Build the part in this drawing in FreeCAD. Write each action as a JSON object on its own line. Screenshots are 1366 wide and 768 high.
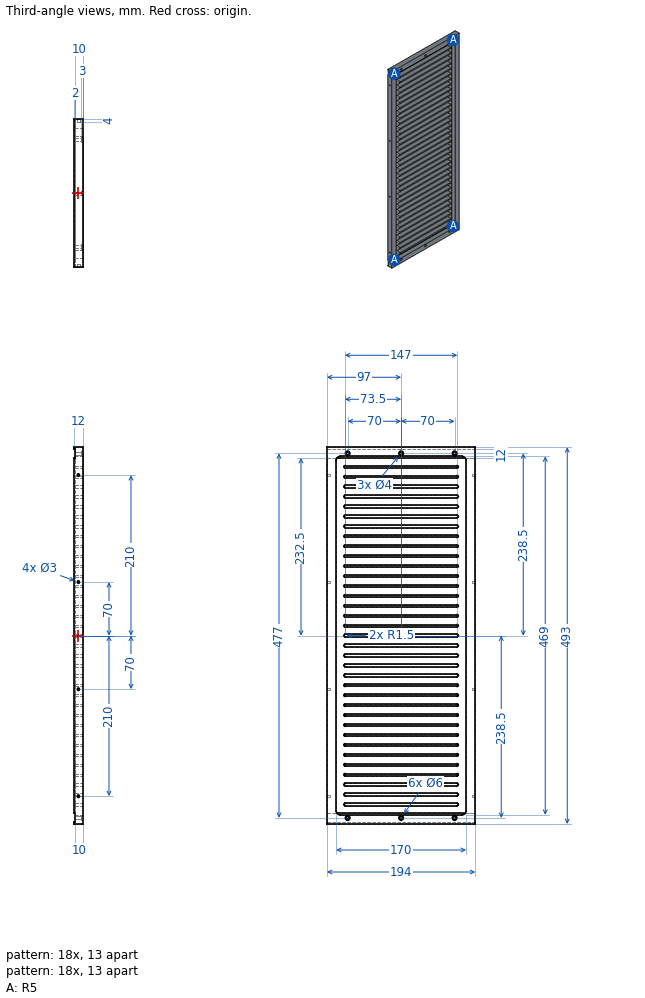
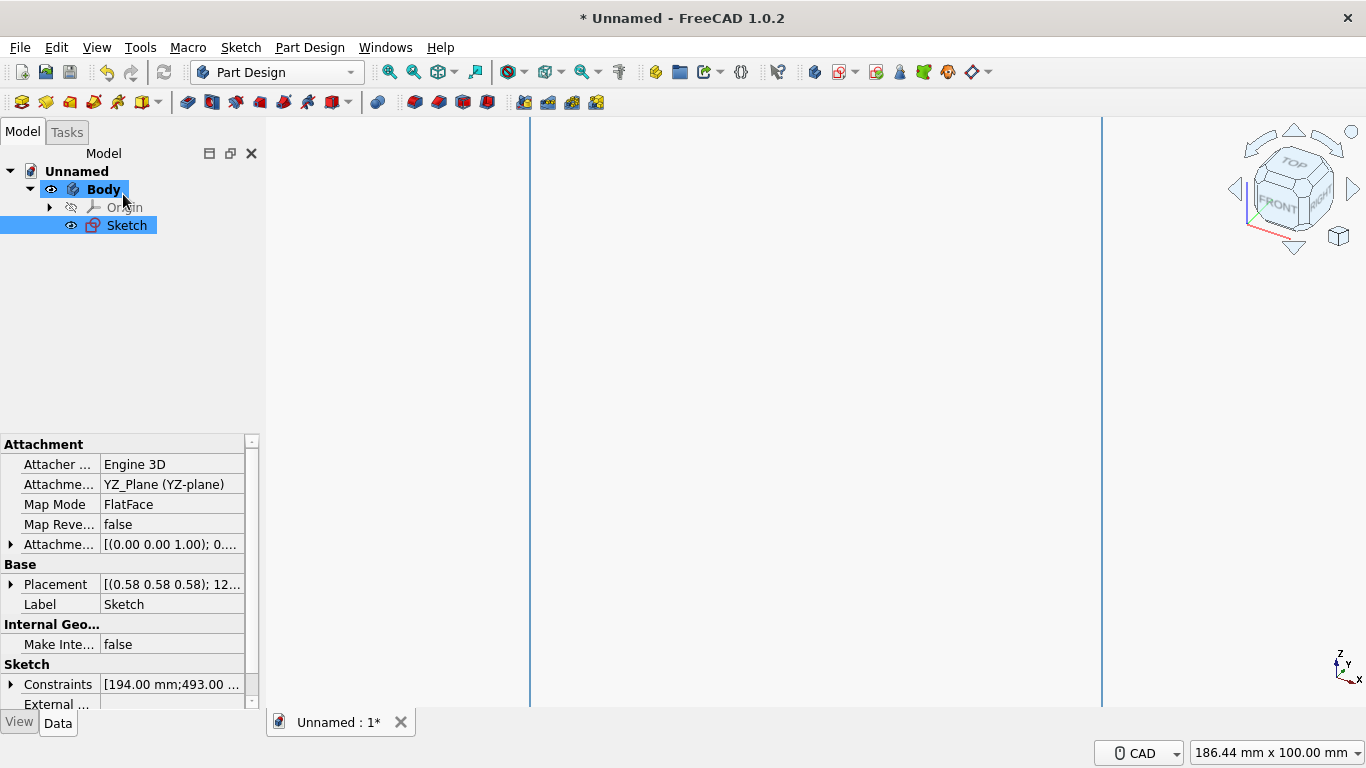
{"action": "left_click", "coordinate": [22, 102]}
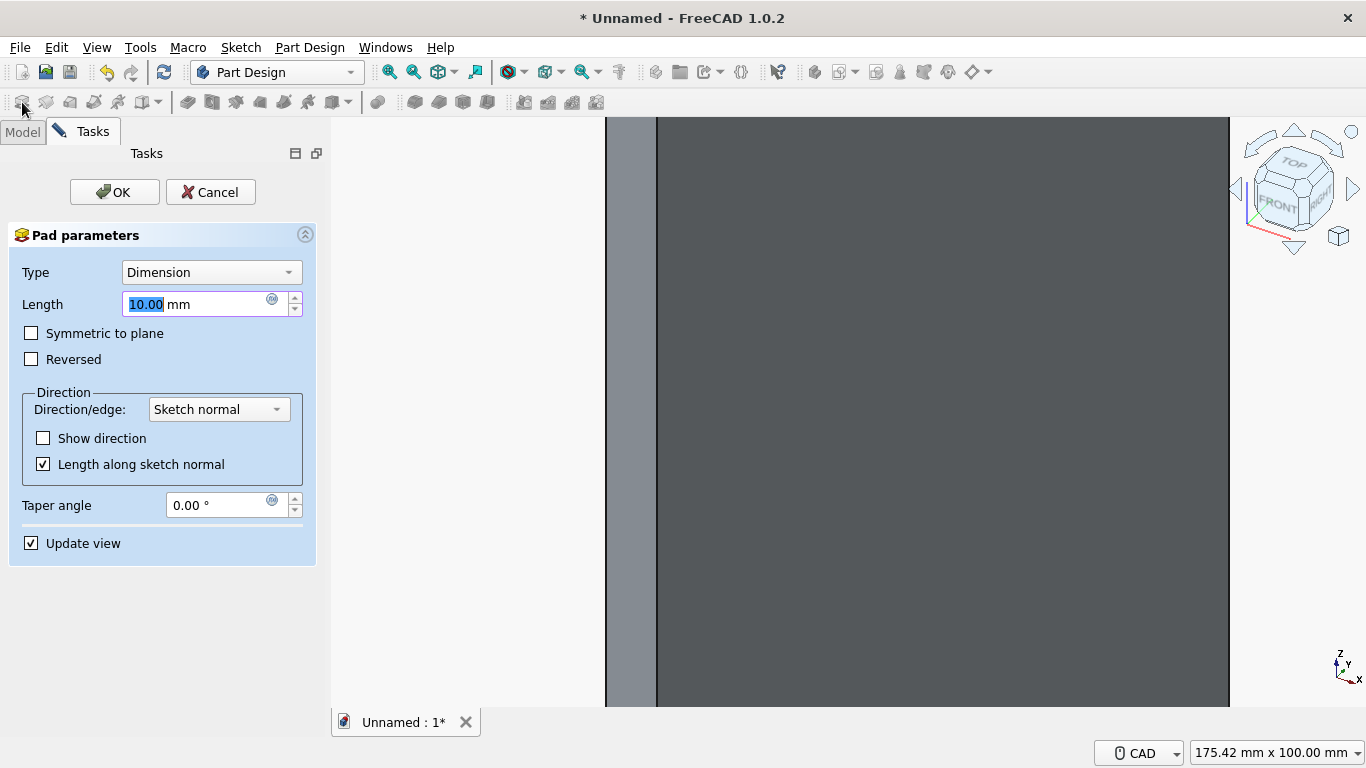
{"action": "type", "text": "12"}
{"action": "key", "text": "Tab"}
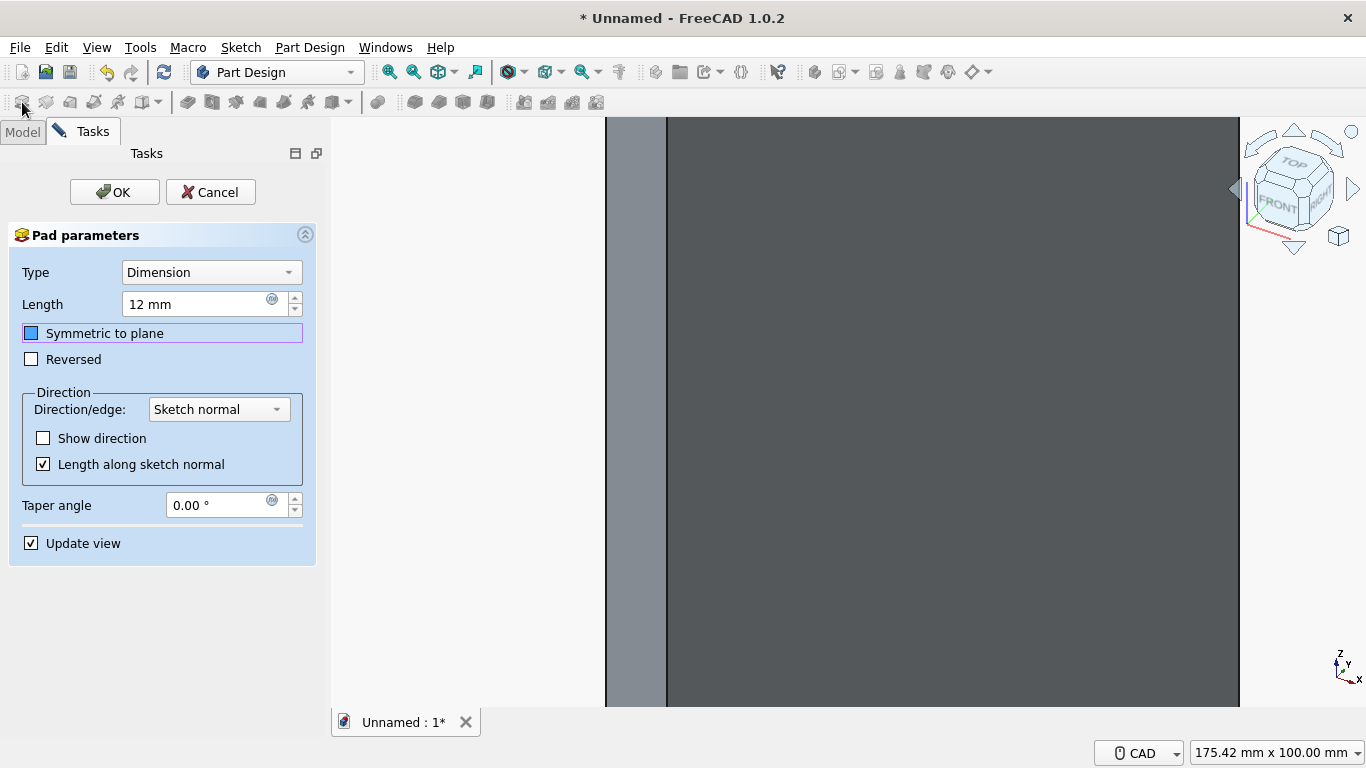
{"action": "left_click", "coordinate": [30, 333]}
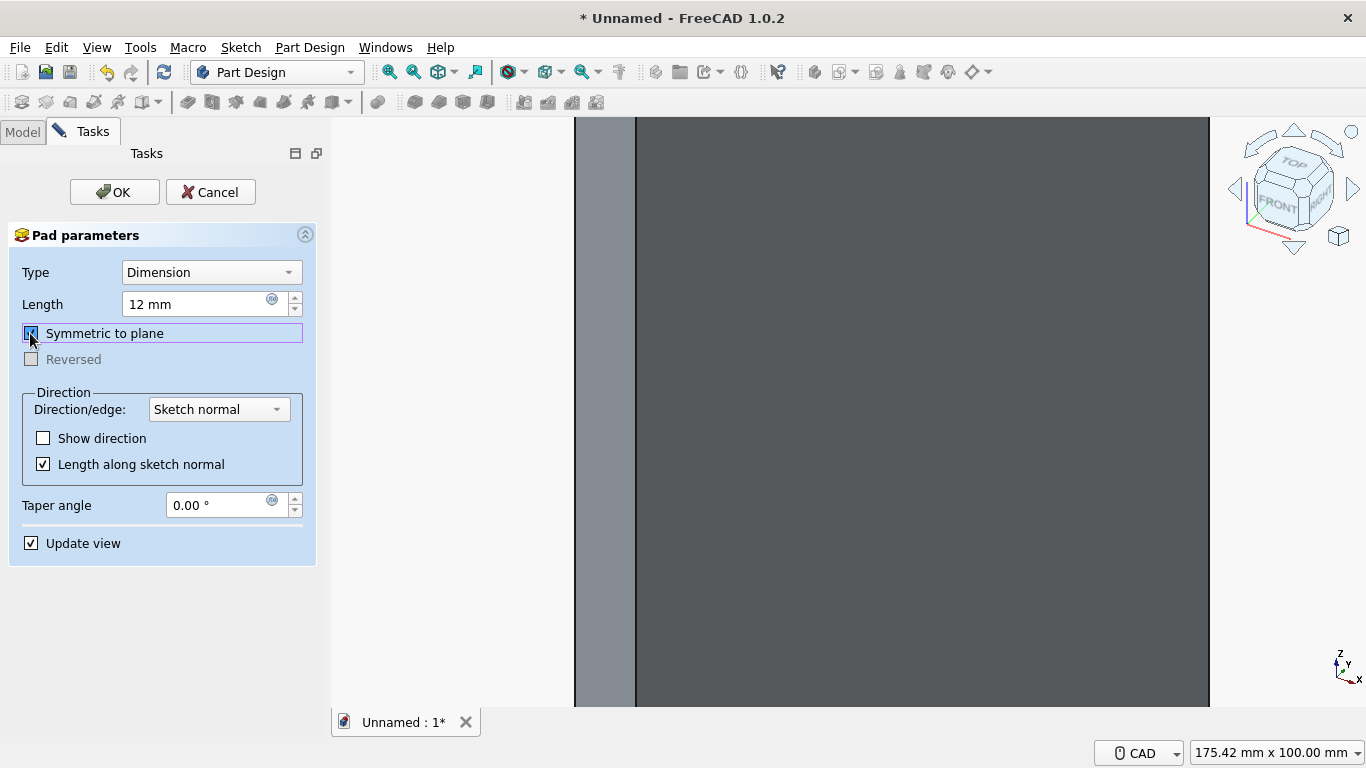
{"action": "left_click", "coordinate": [115, 192]}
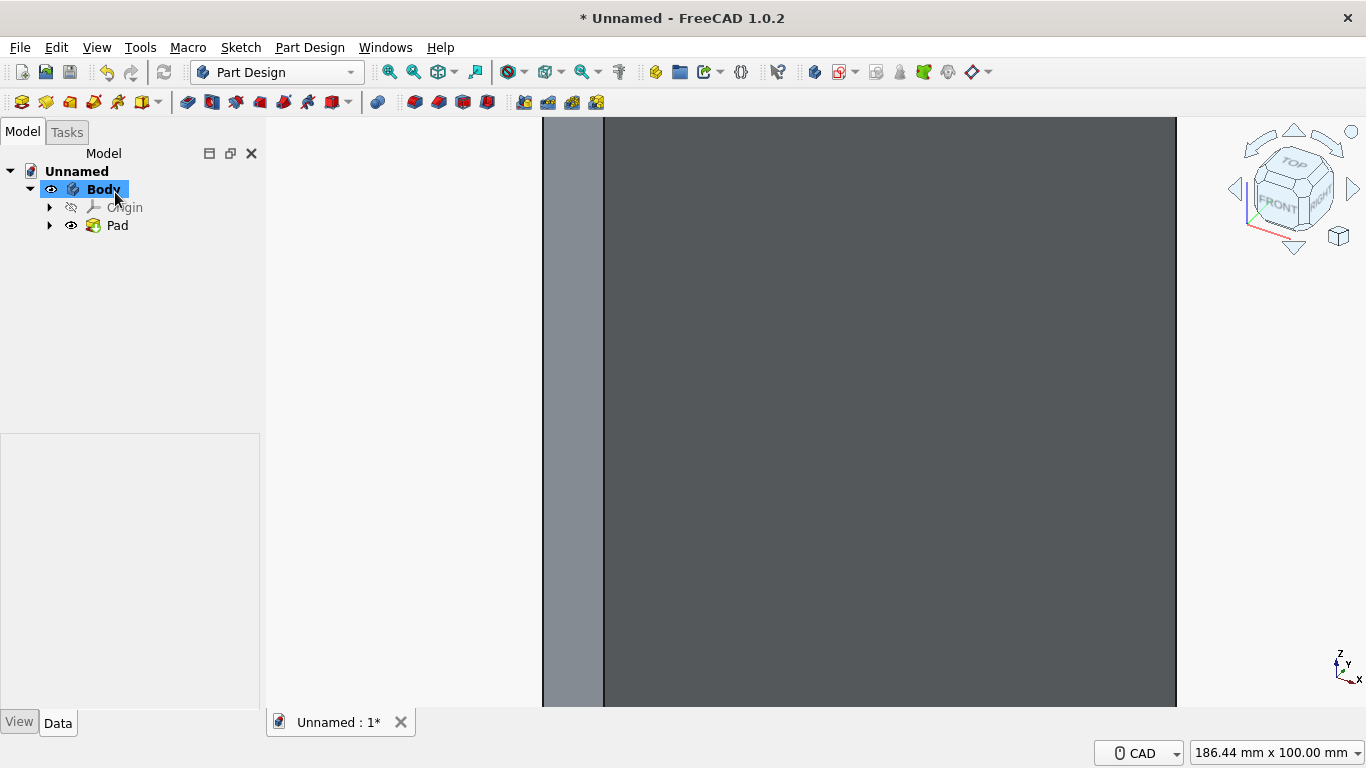
{"action": "left_click", "coordinate": [390, 72]}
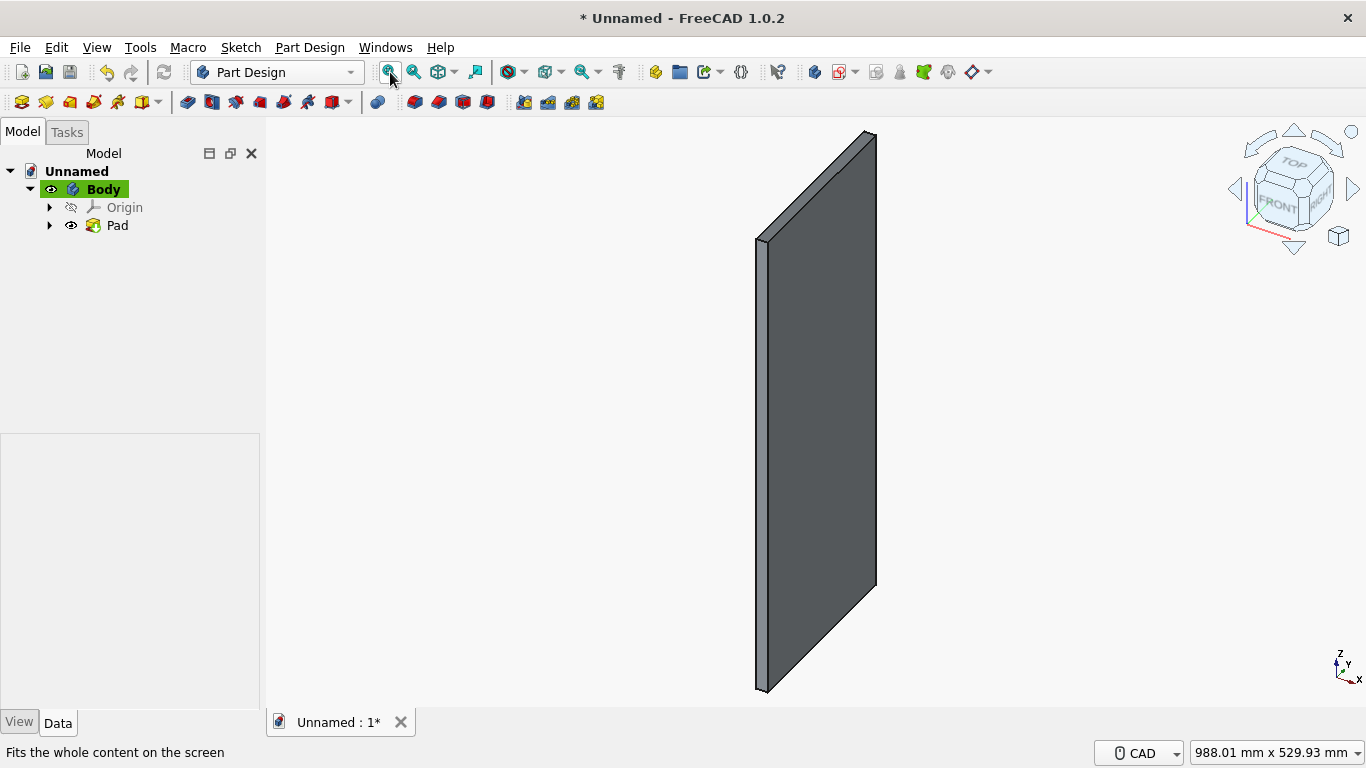
{"action": "left_click", "coordinate": [822, 541]}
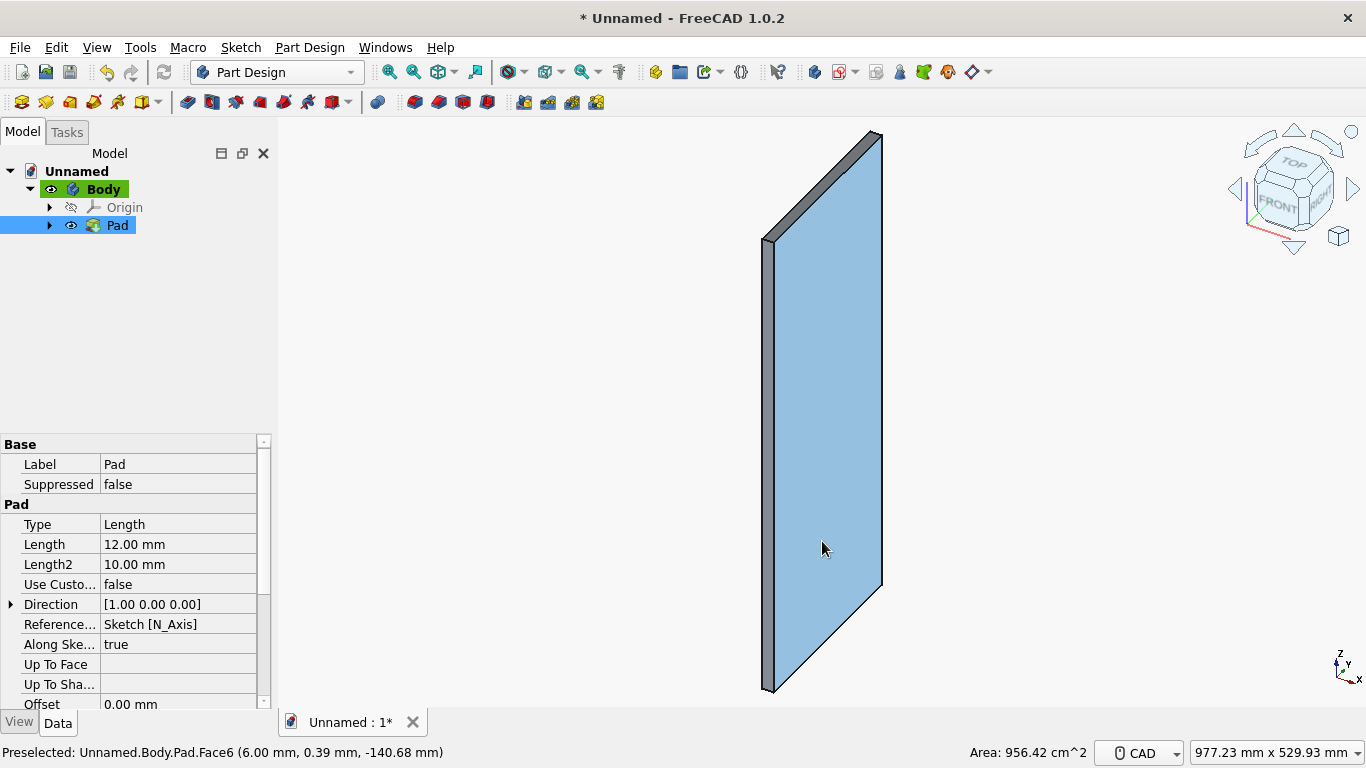
{"action": "left_click", "coordinate": [840, 72]}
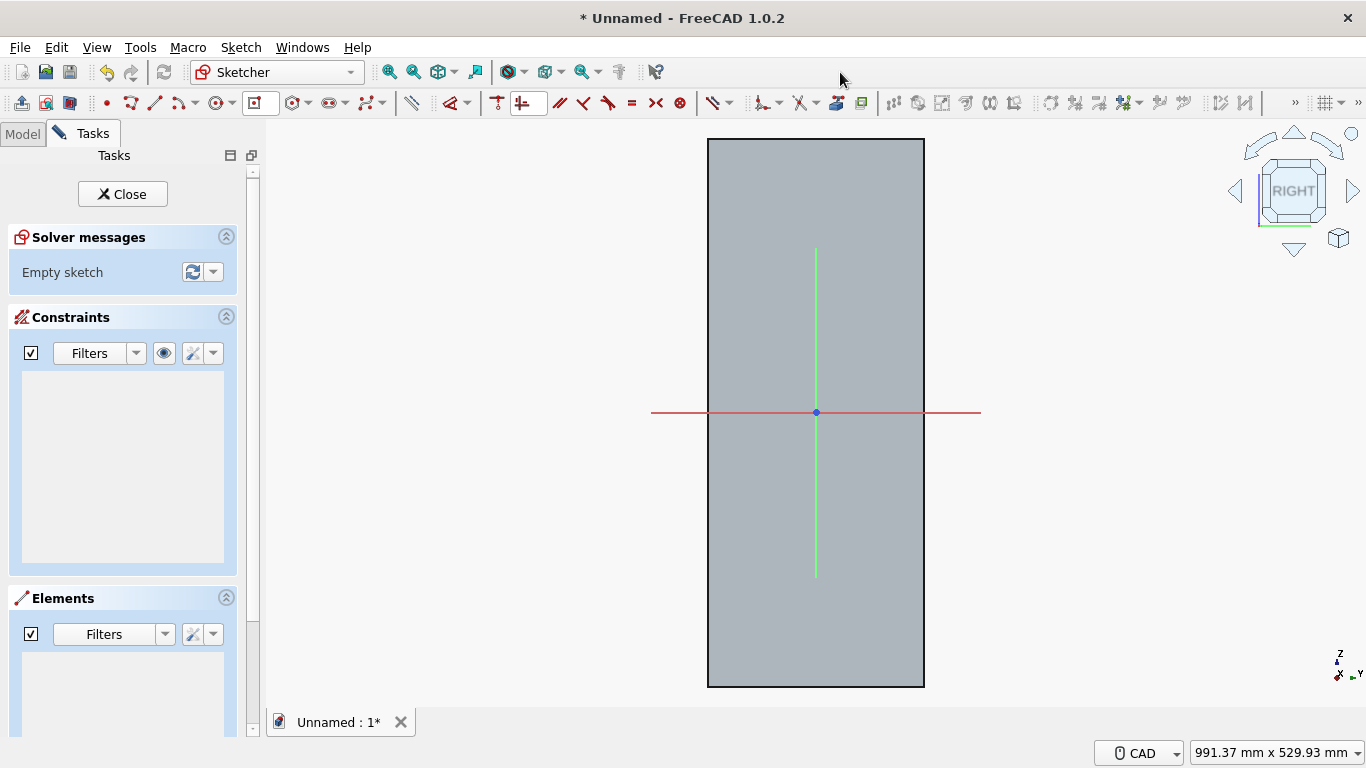
{"action": "scroll", "coordinate": [608, 413], "scroll_direction": "down", "scroll_amount": 2}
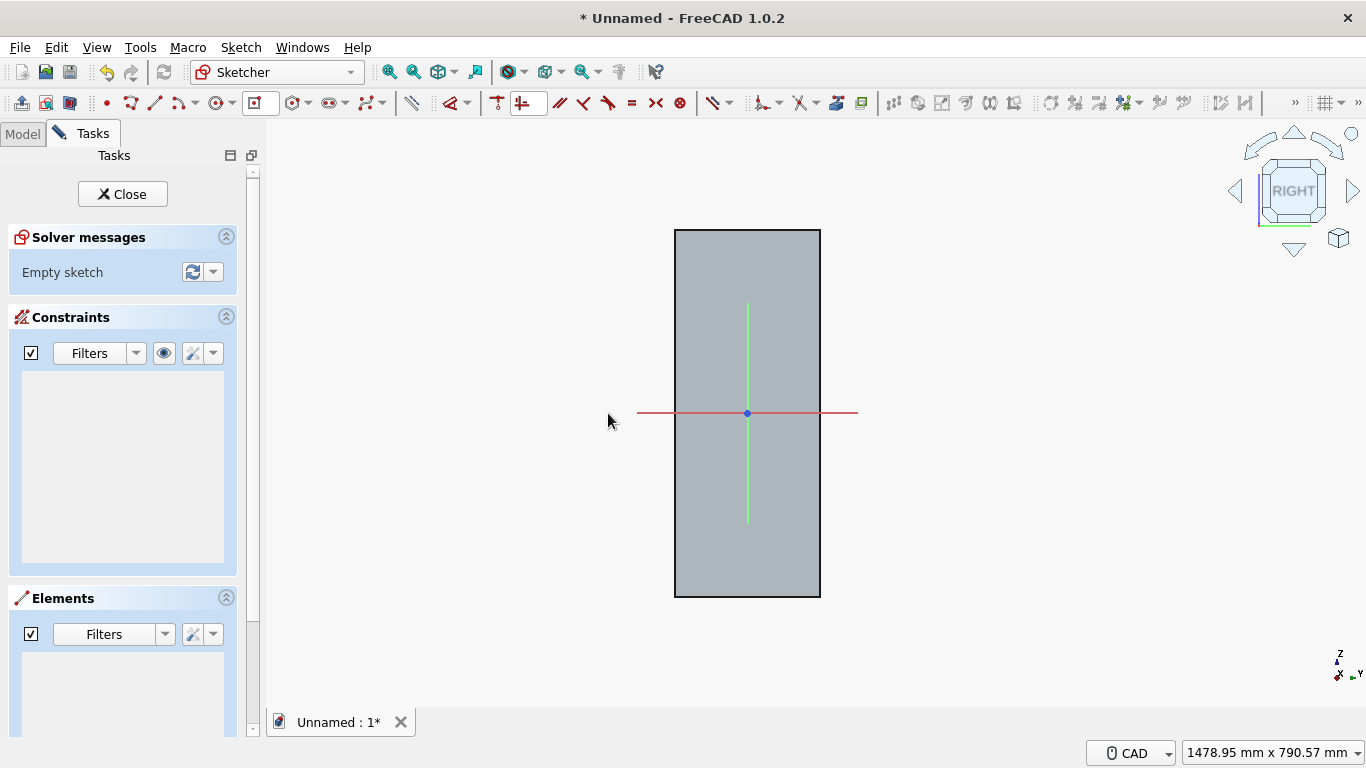
{"action": "left_click", "coordinate": [254, 104]}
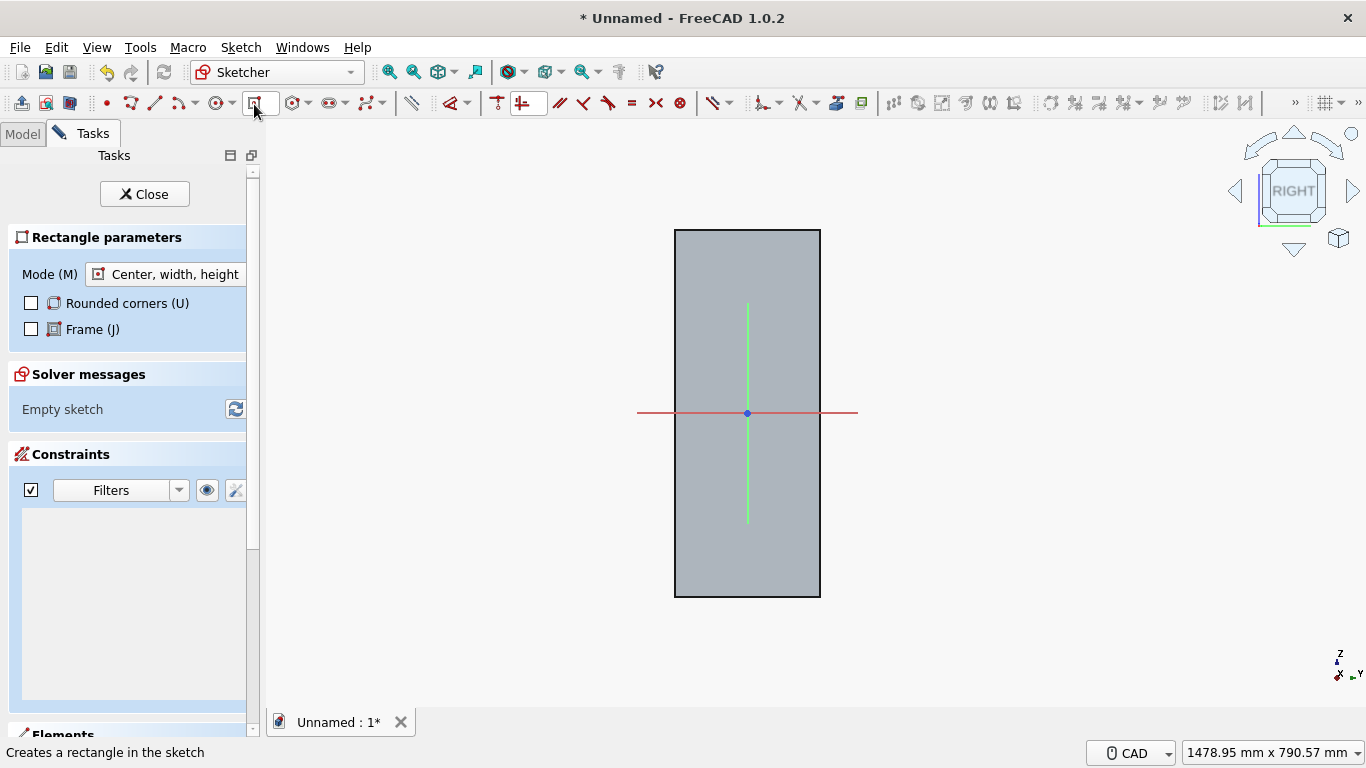
{"action": "left_click", "coordinate": [748, 413]}
{"action": "mouse_move", "coordinate": [811, 239]}